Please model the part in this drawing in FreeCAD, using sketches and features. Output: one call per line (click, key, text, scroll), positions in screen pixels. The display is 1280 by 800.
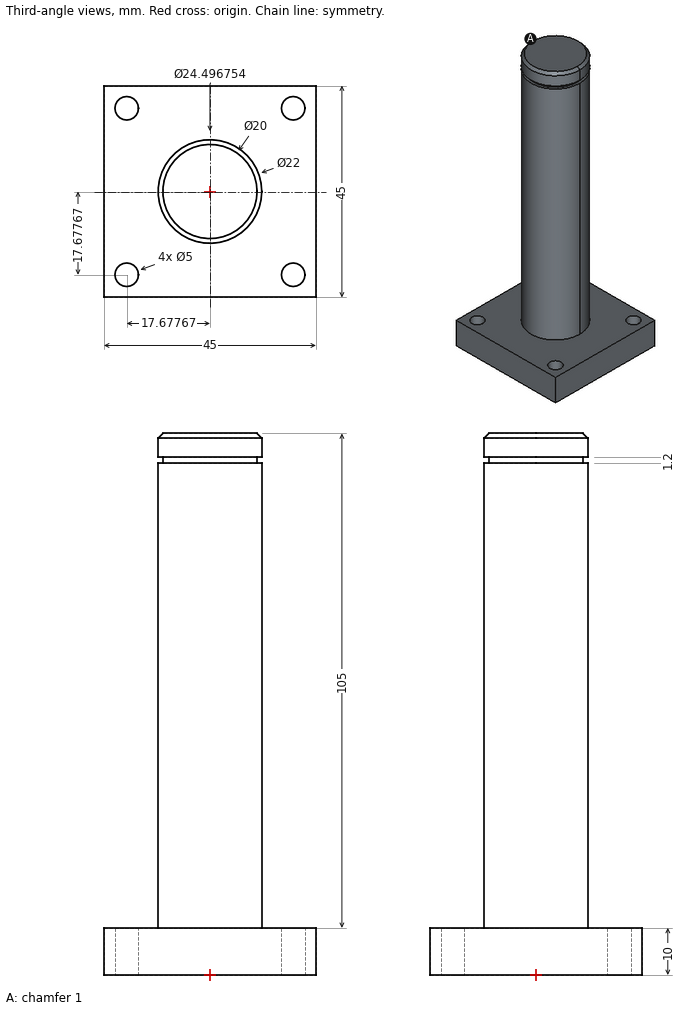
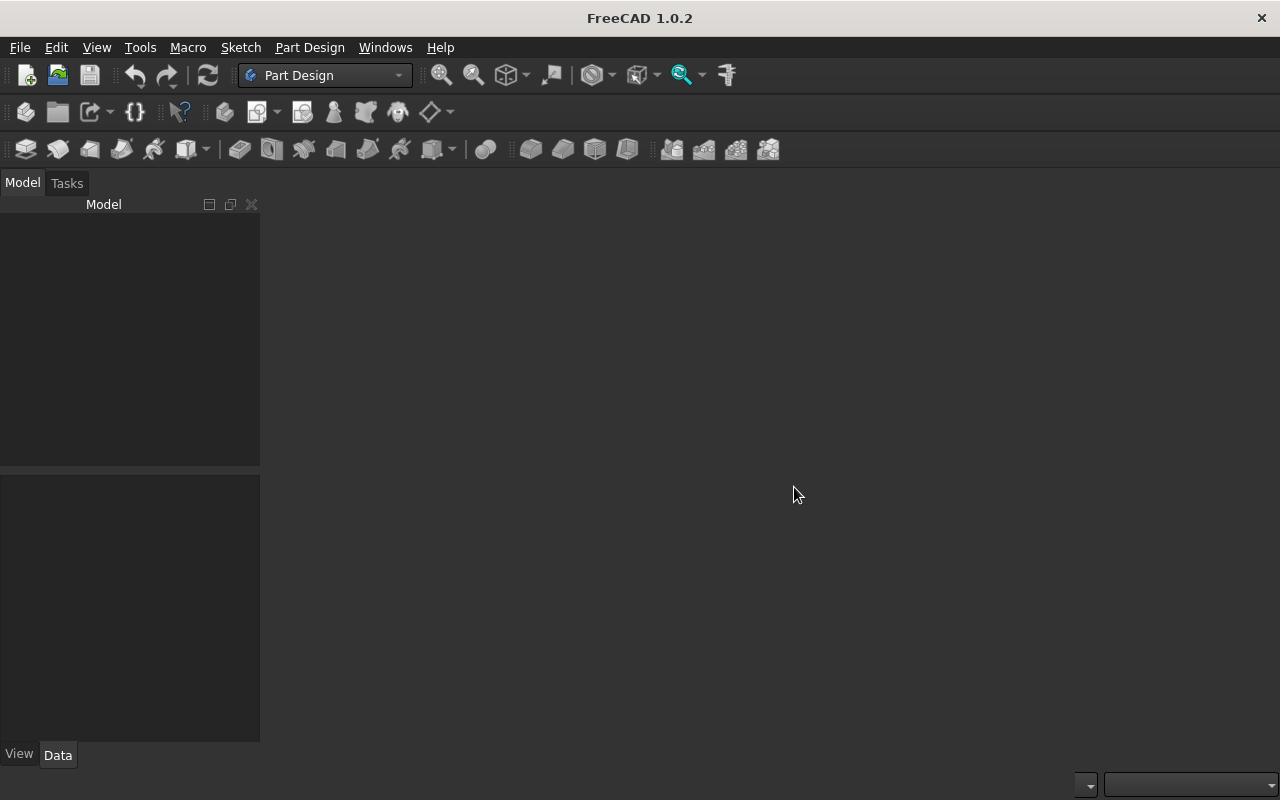
click(26, 76)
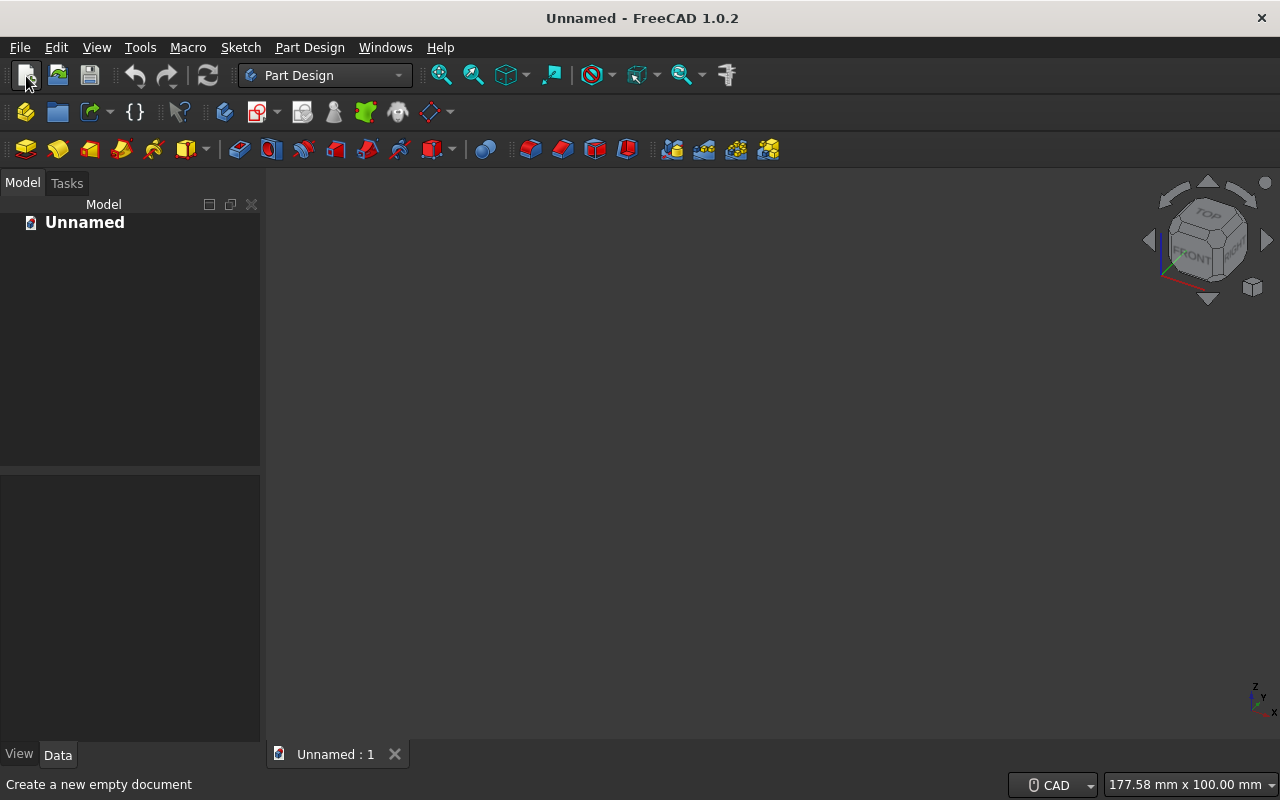
click(258, 112)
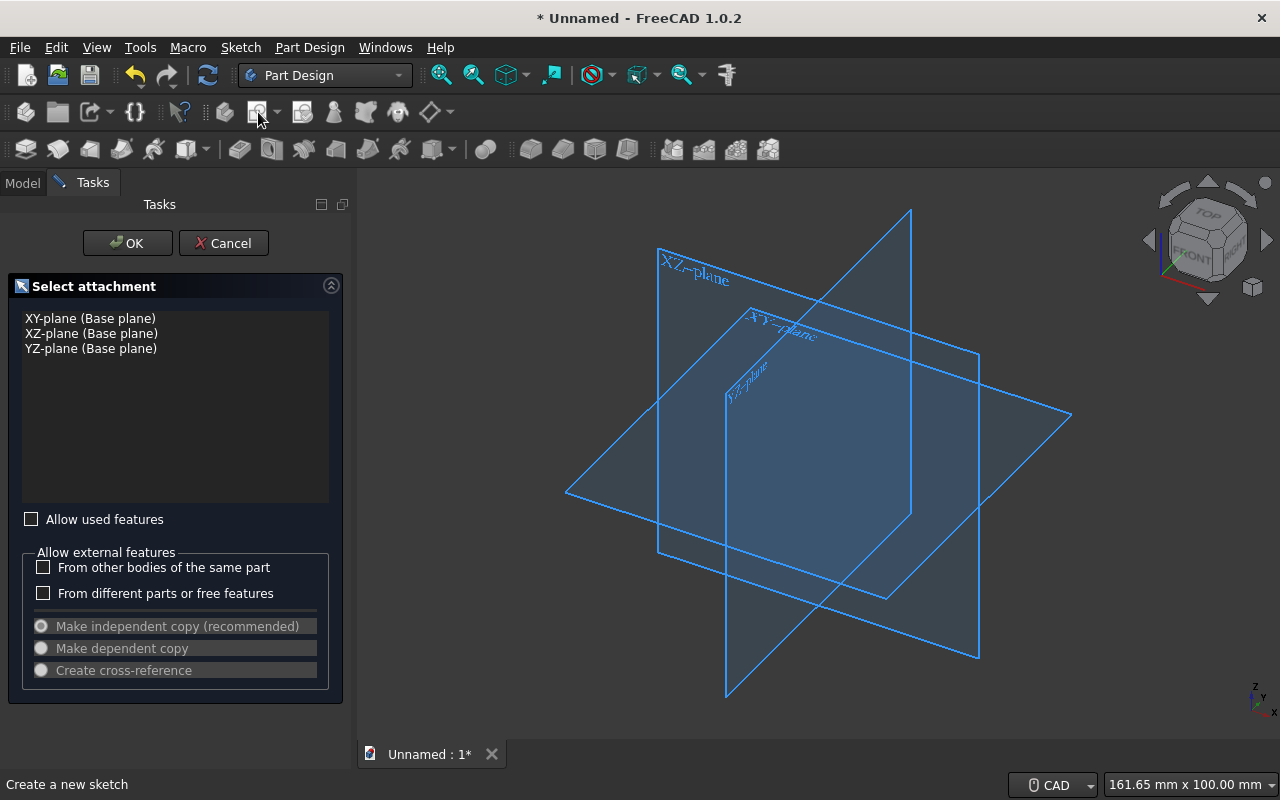
click(82, 318)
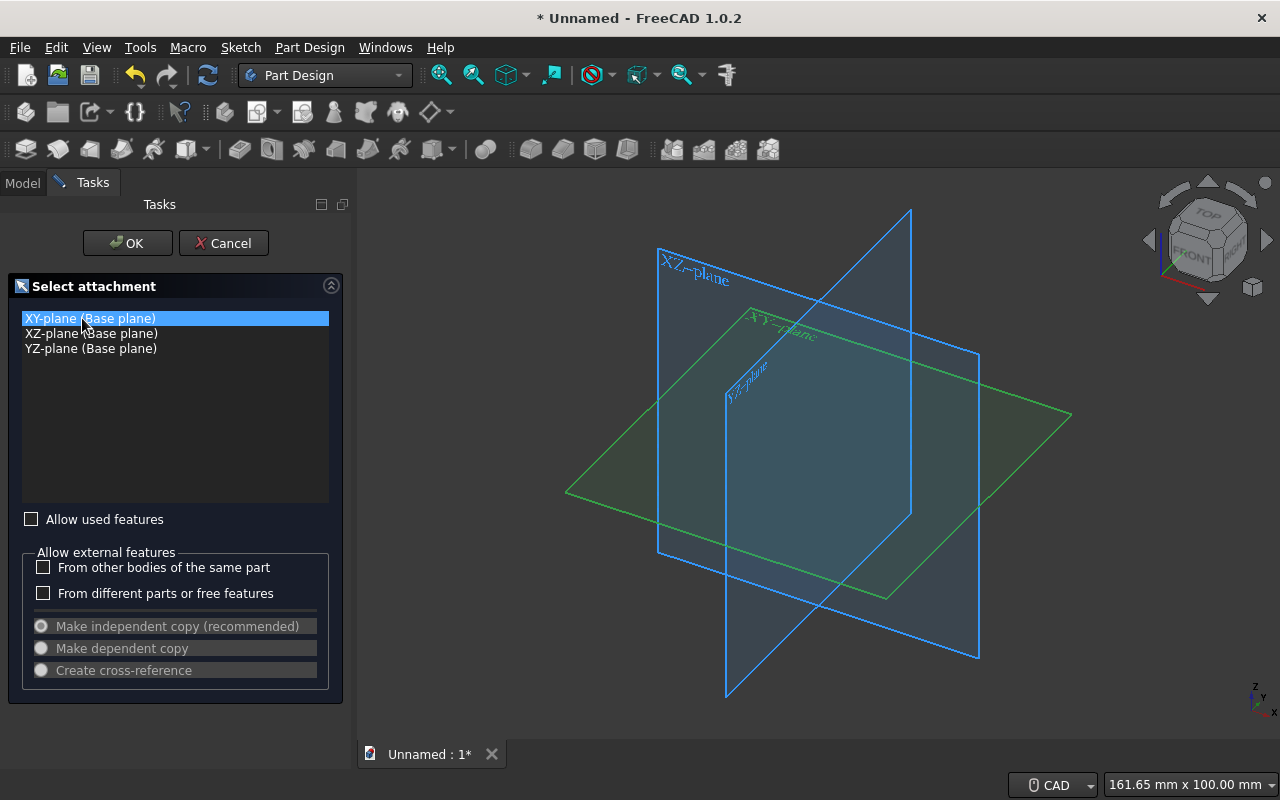
click(128, 243)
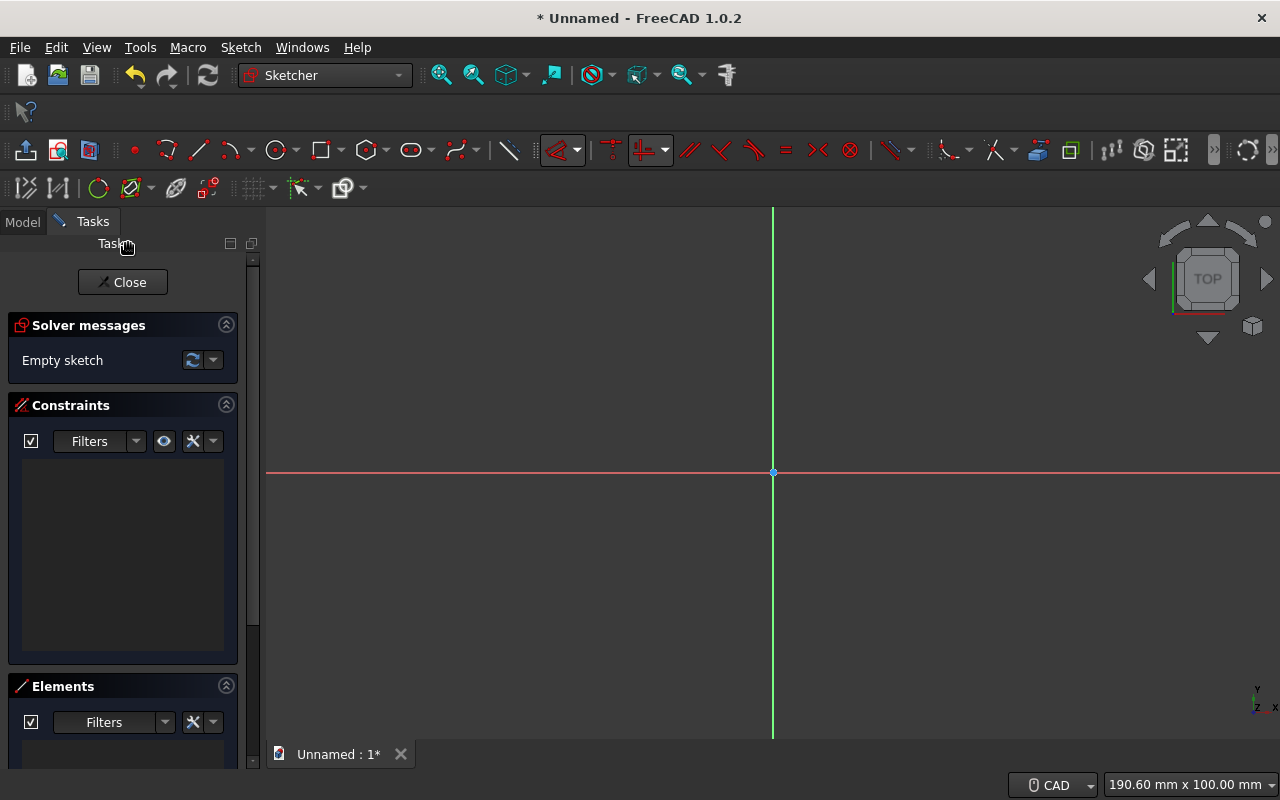
scroll(912, 473, up, 2)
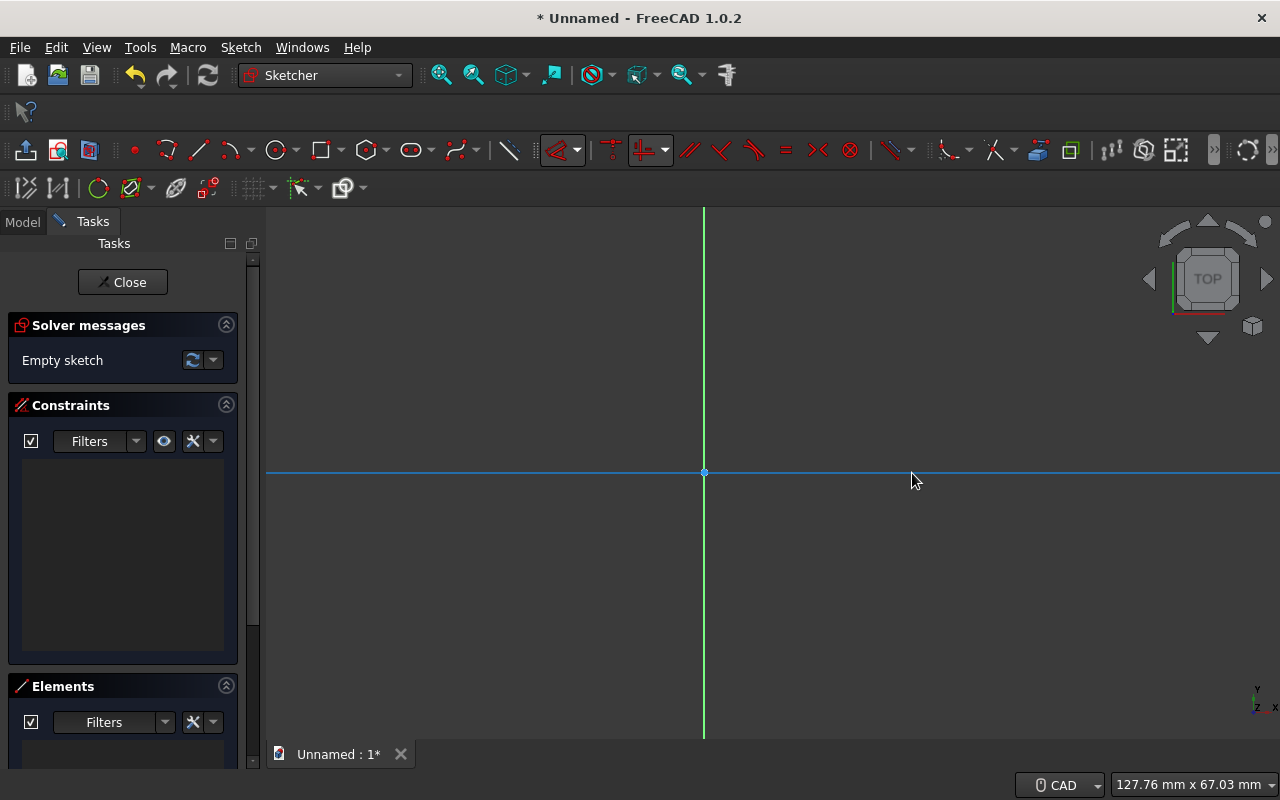
click(344, 150)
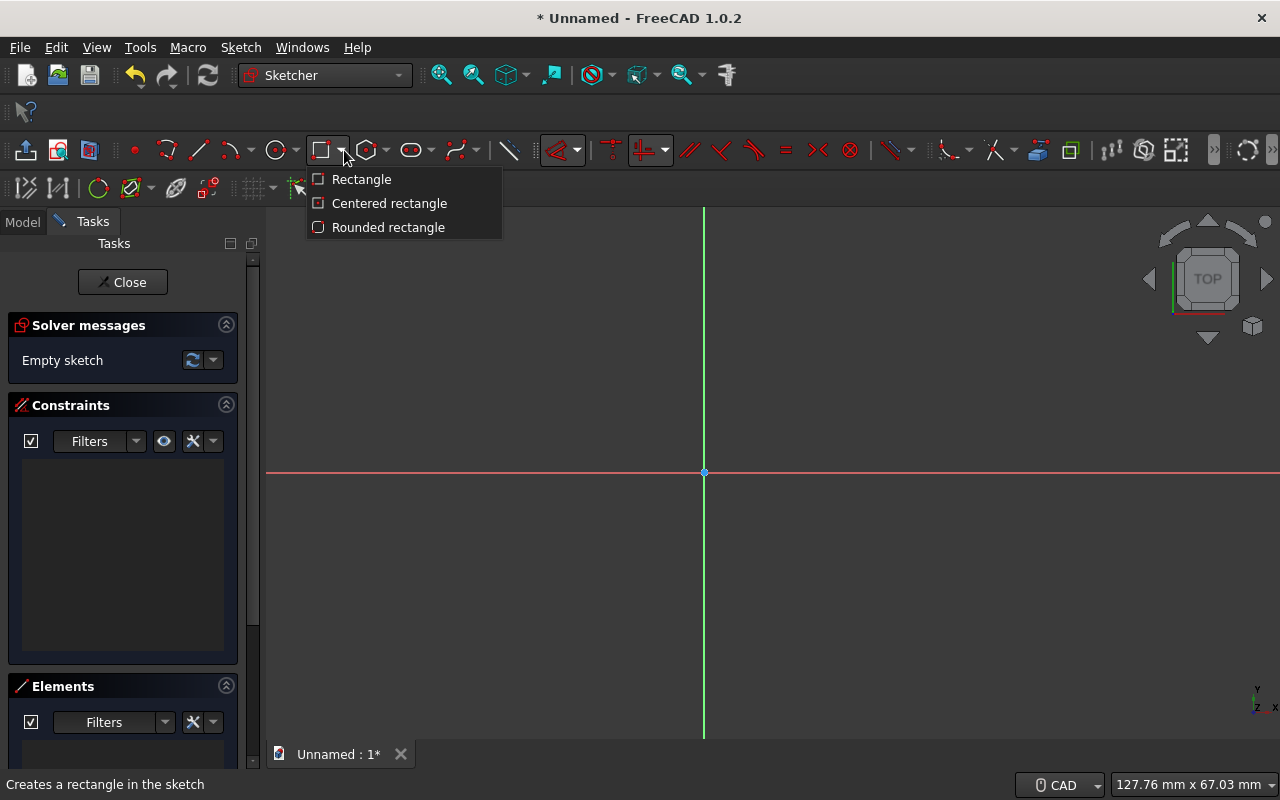
click(404, 203)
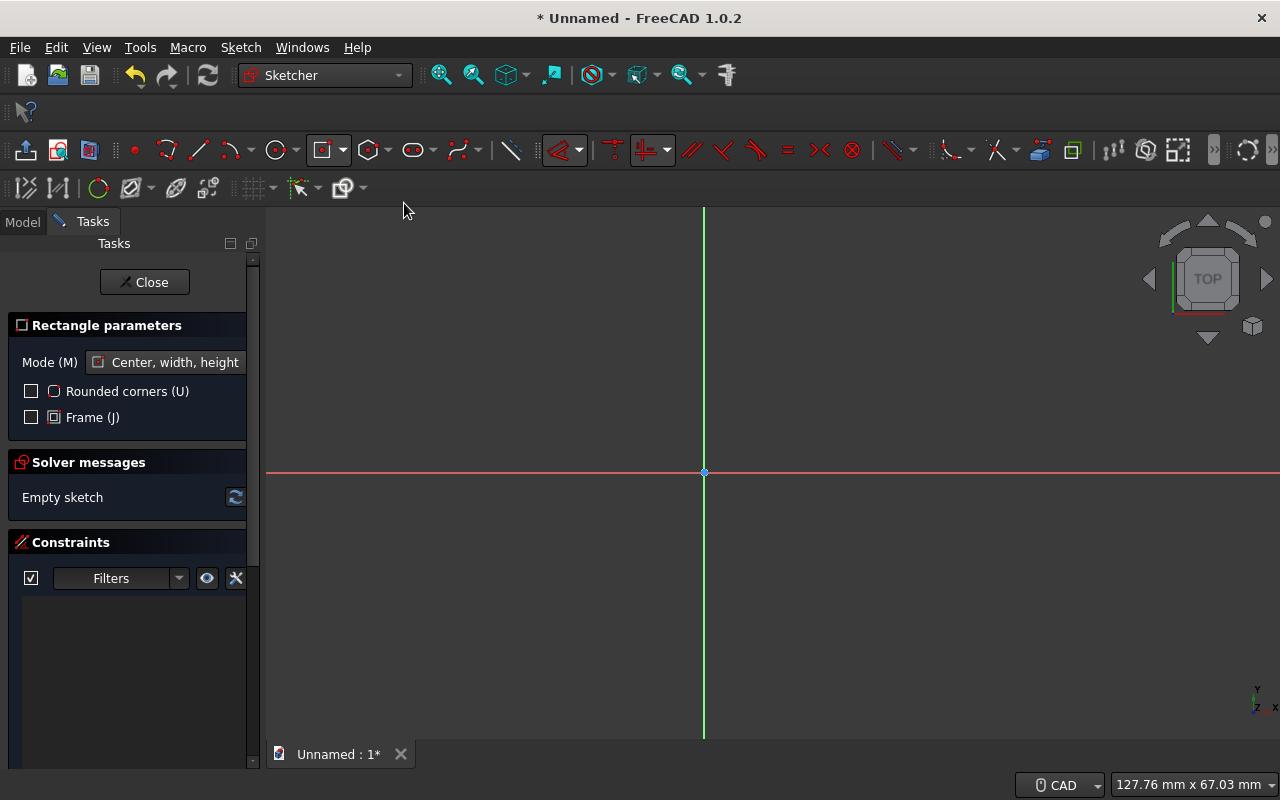
click(704, 473)
move(883, 294)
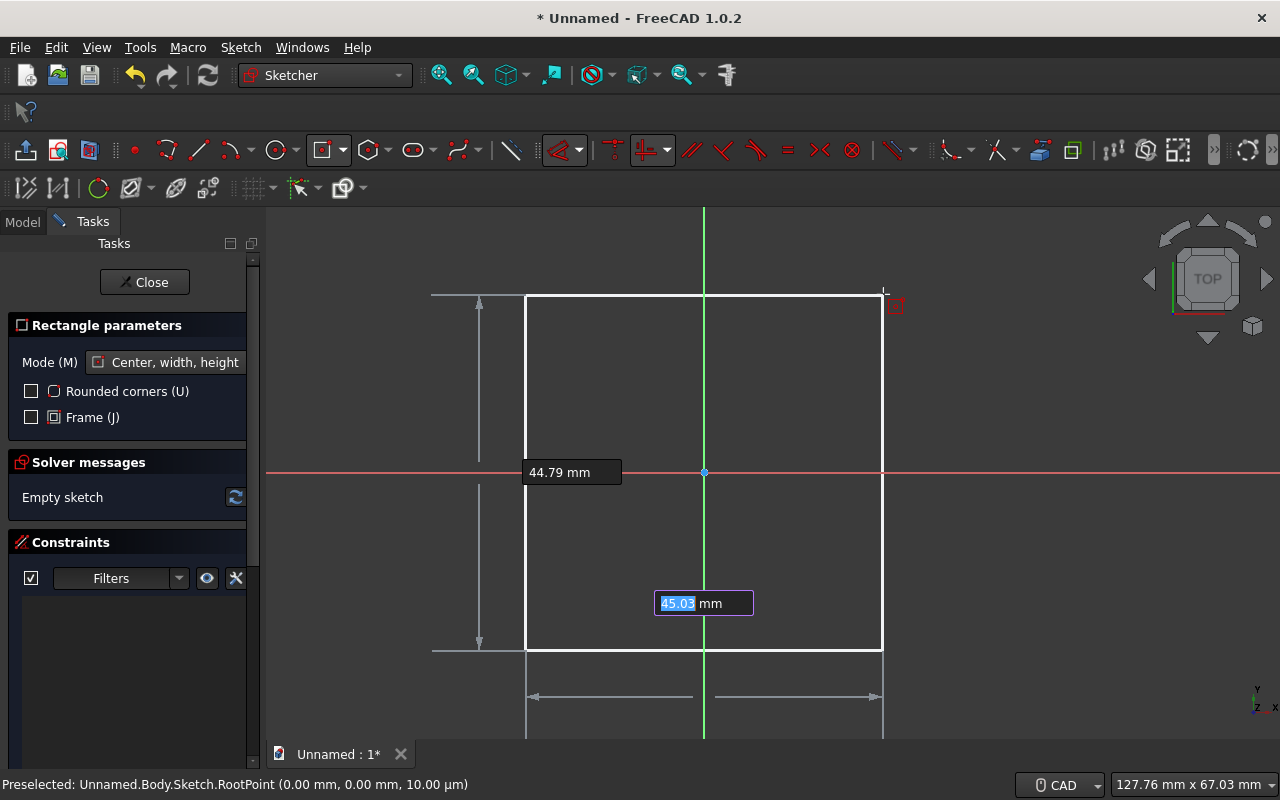
text(45)
key(Tab)
text(45)
key(Return)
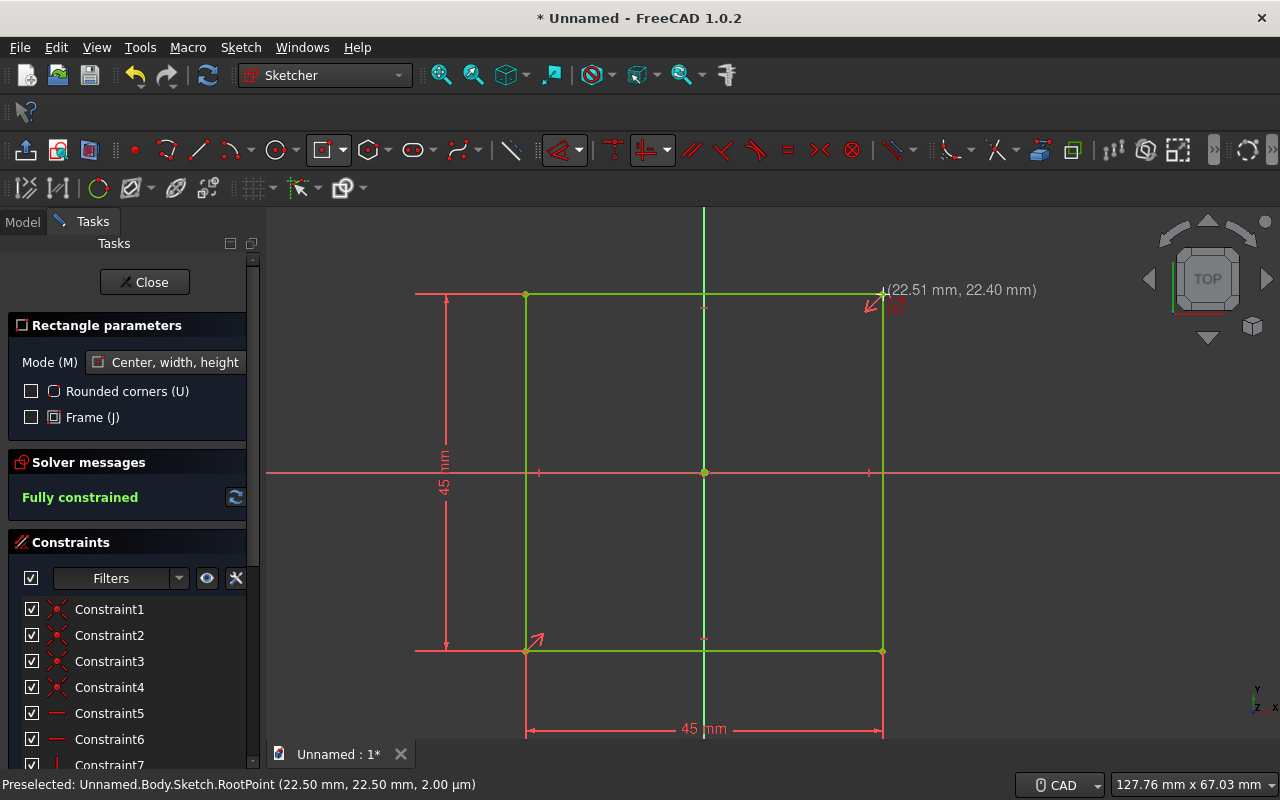
click(276, 150)